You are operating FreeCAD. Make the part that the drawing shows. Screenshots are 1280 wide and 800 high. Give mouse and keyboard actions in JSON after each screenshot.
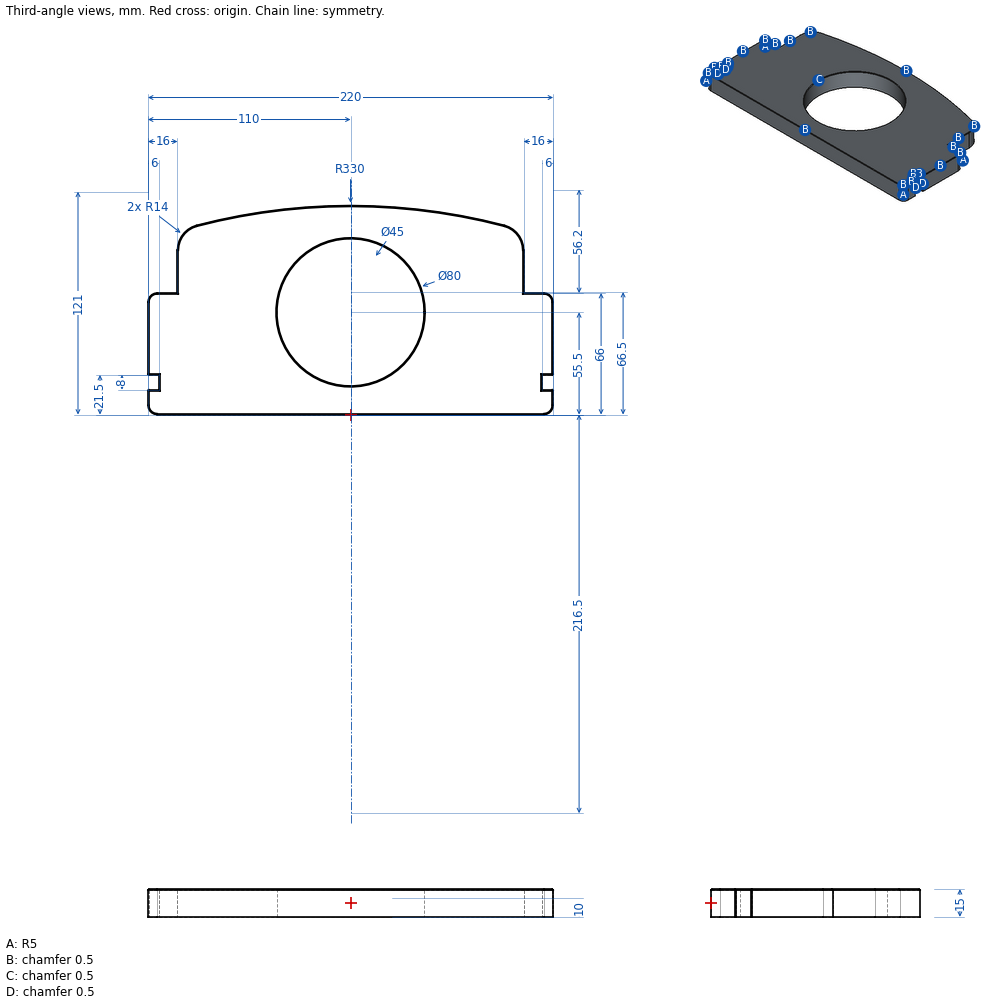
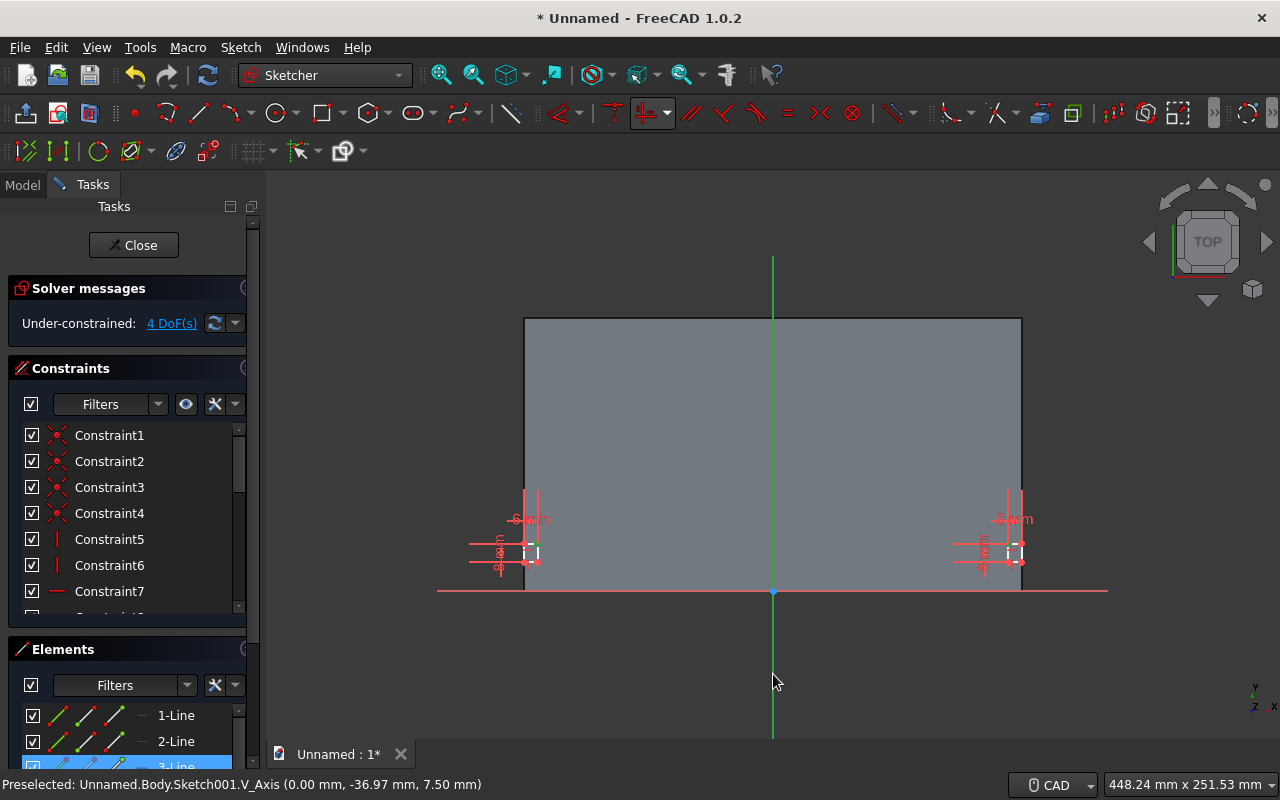
{"action": "left_click", "coordinate": [820, 114]}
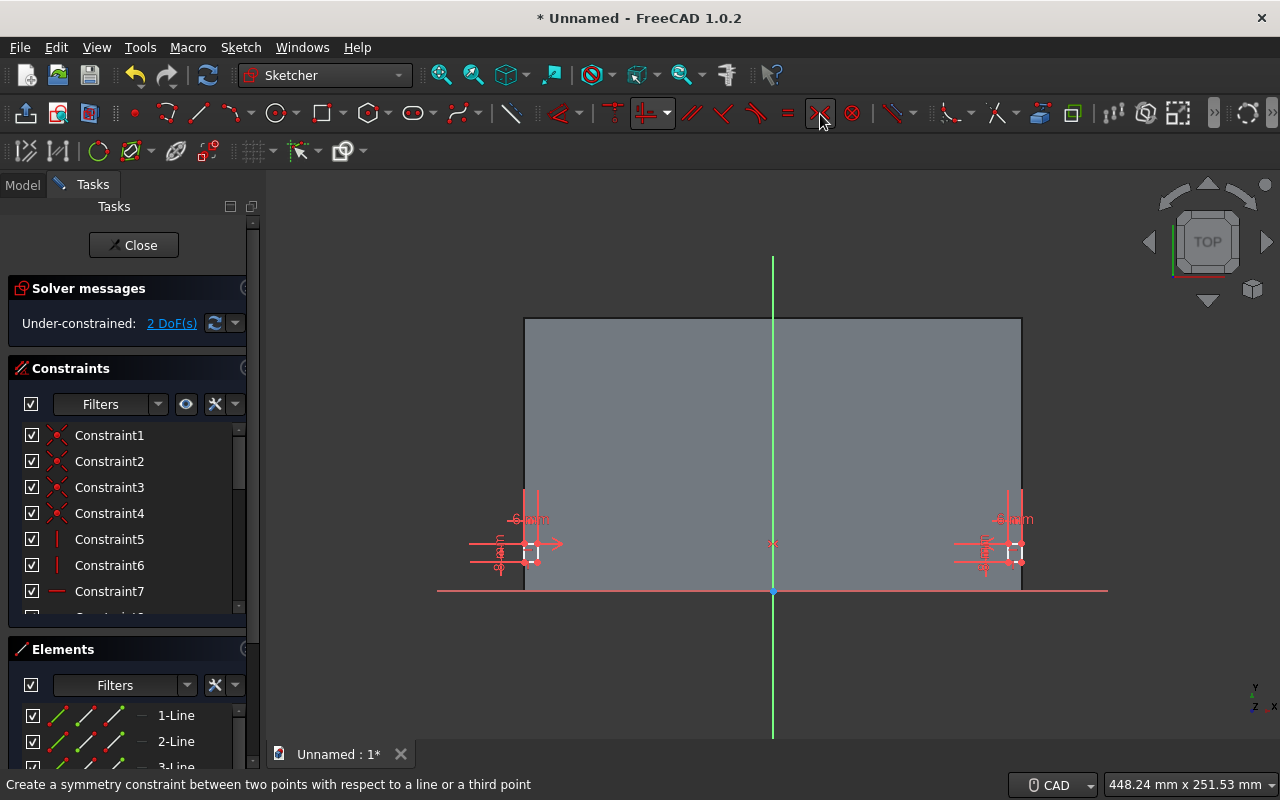
{"action": "left_click", "coordinate": [558, 114]}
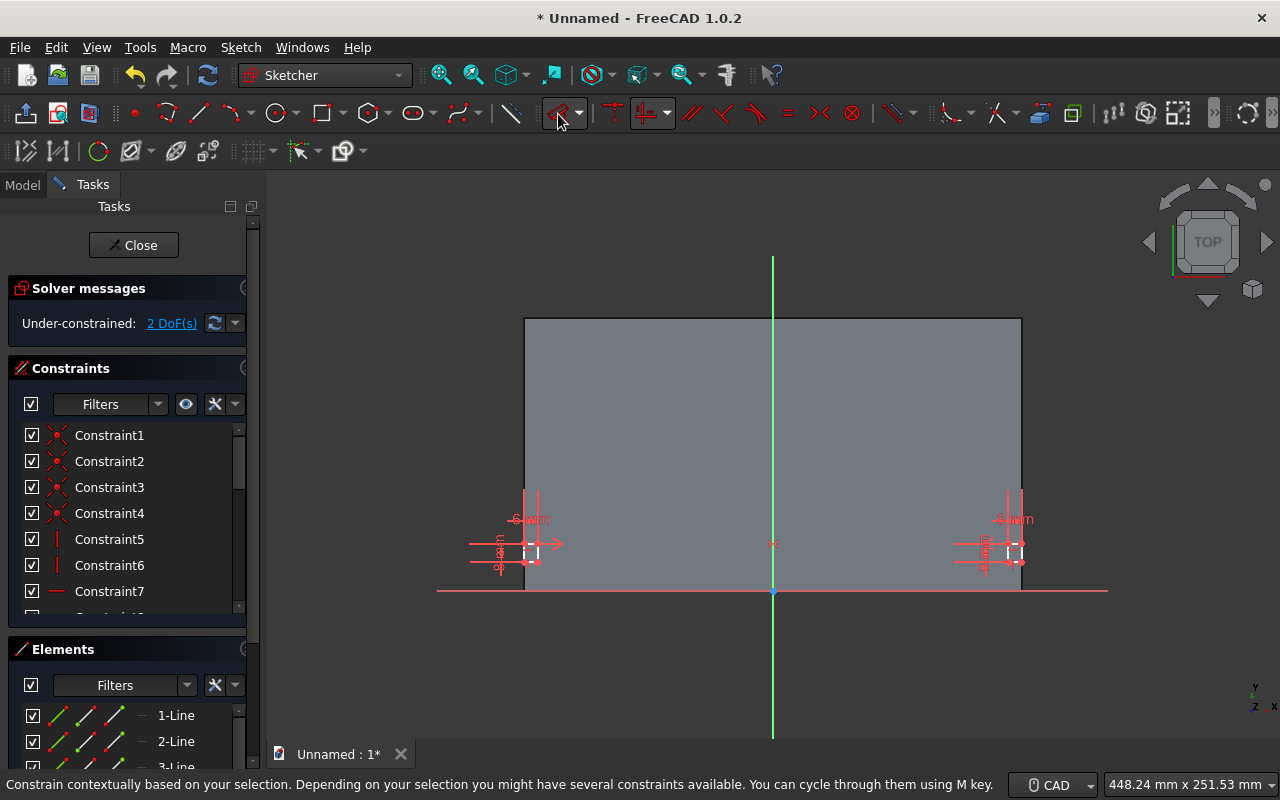
{"action": "left_click", "coordinate": [524, 544]}
{"action": "left_click", "coordinate": [649, 625]}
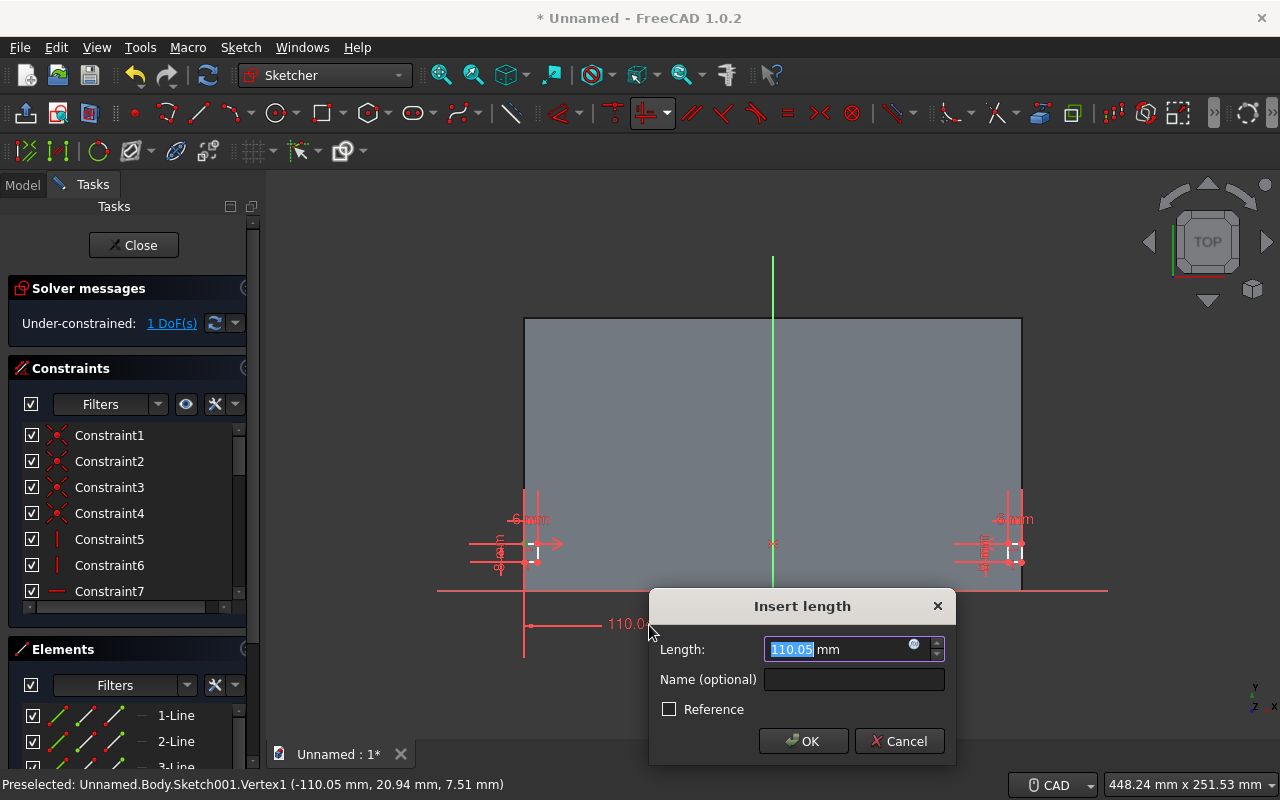
{"action": "type", "text": "110"}
{"action": "key", "text": "Return"}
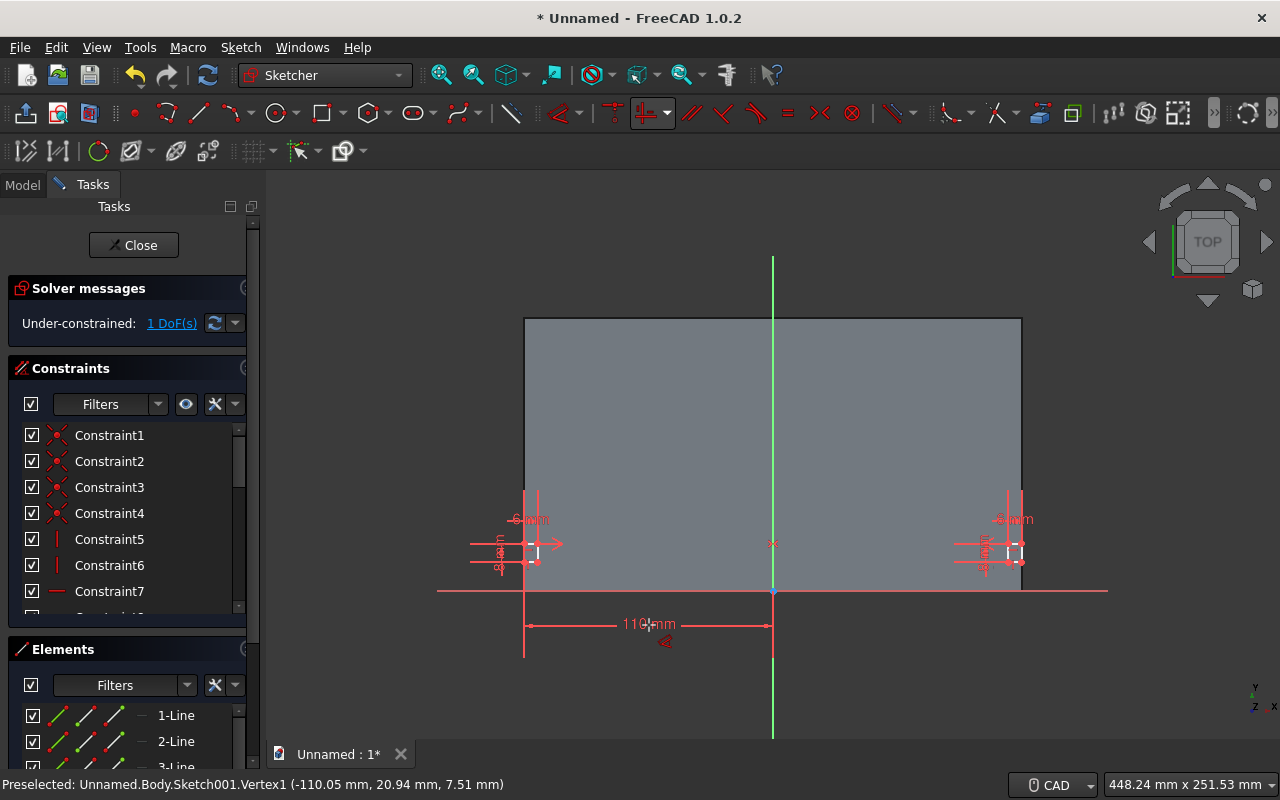
{"action": "left_click", "coordinate": [524, 544]}
{"action": "left_click", "coordinate": [490, 568]}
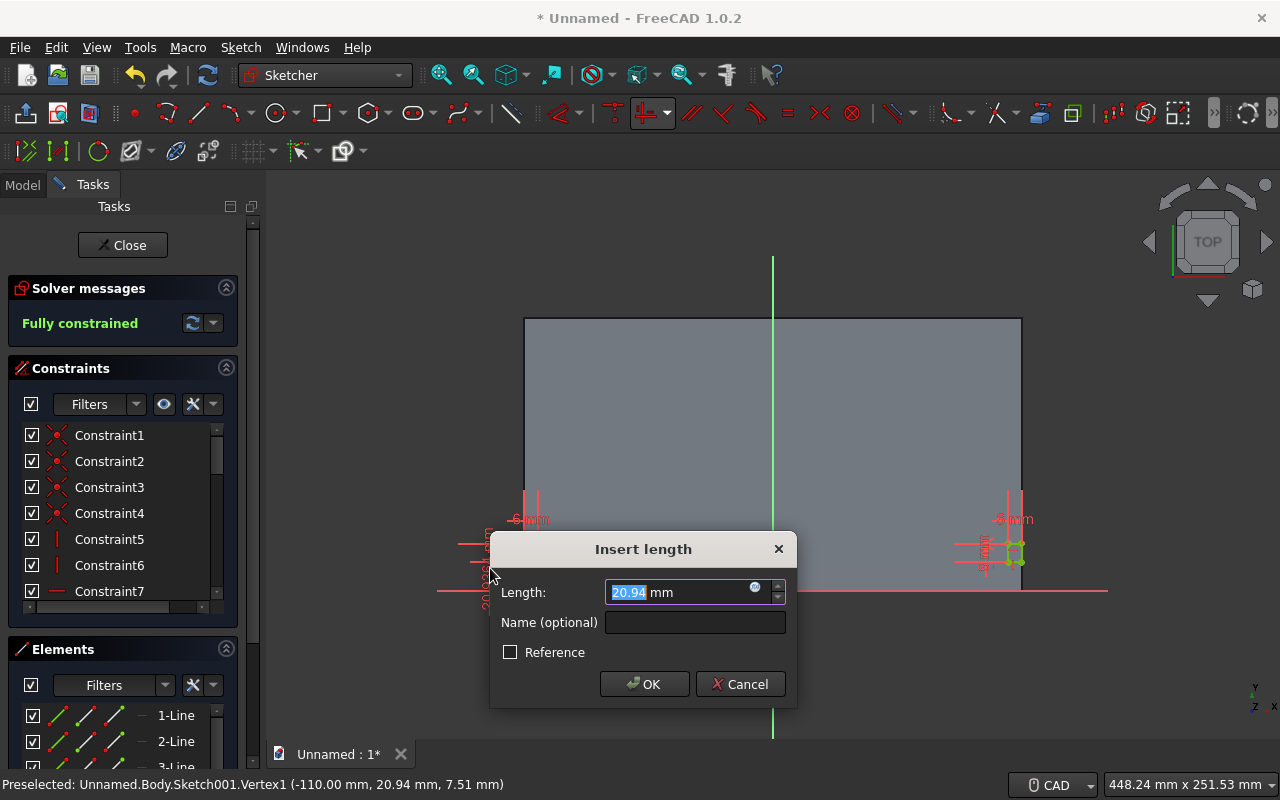
{"action": "type", "text": "21.5"}
{"action": "key", "text": "Return"}
{"action": "key", "text": "Escape"}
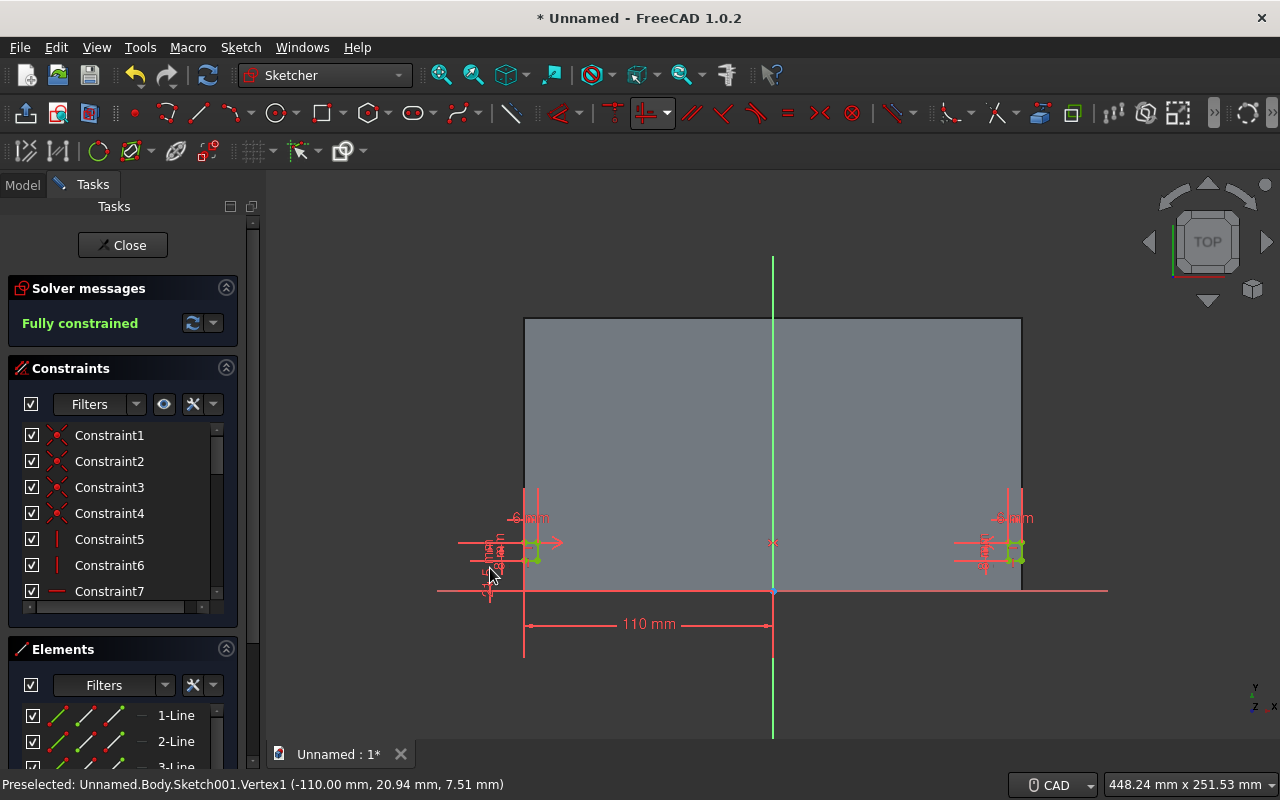
{"action": "left_click", "coordinate": [123, 245]}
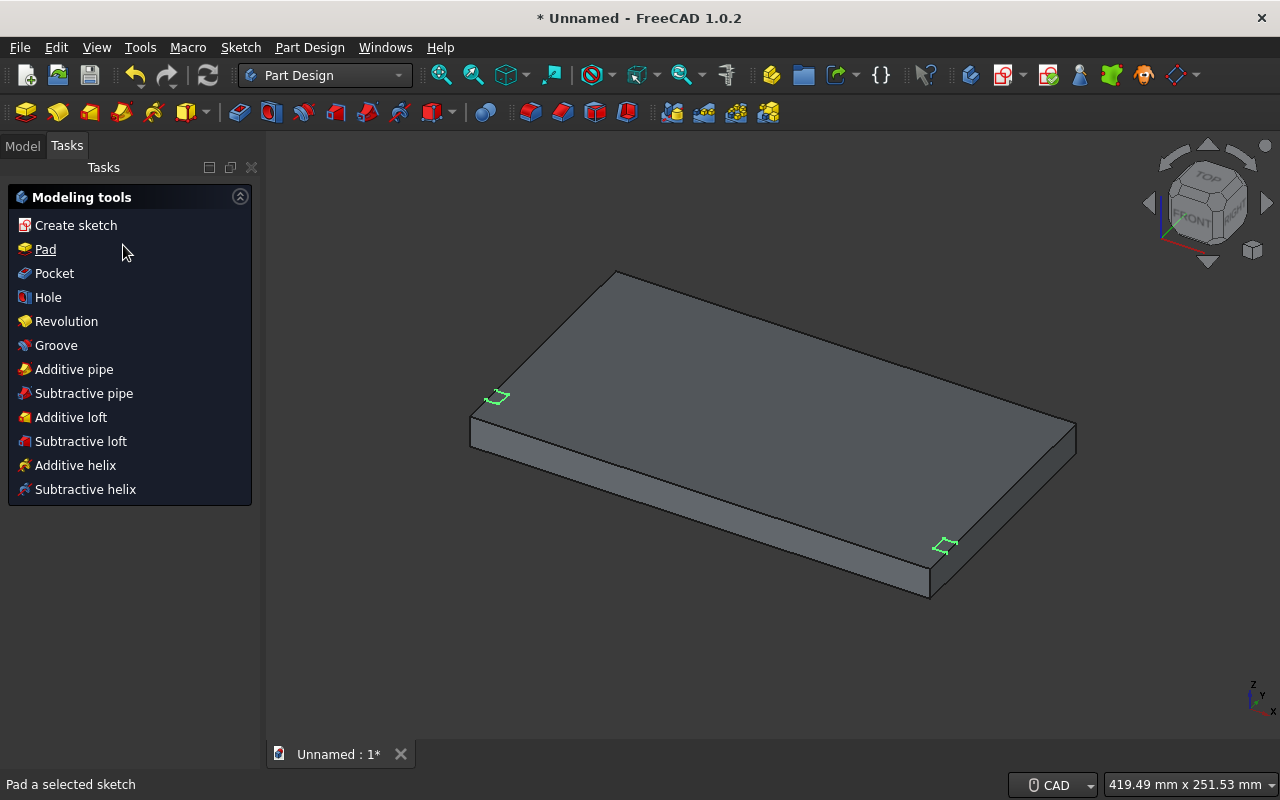
{"action": "left_click", "coordinate": [240, 112]}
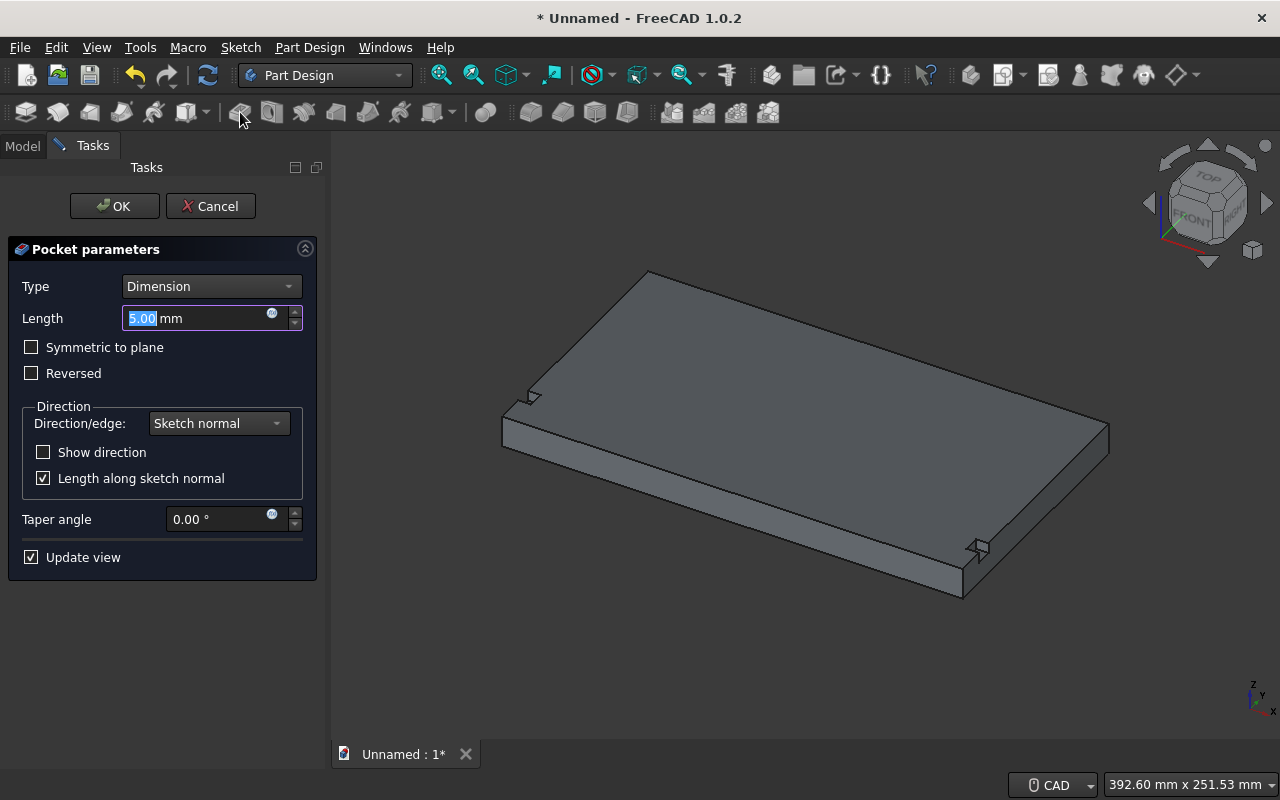
{"action": "left_click", "coordinate": [212, 286]}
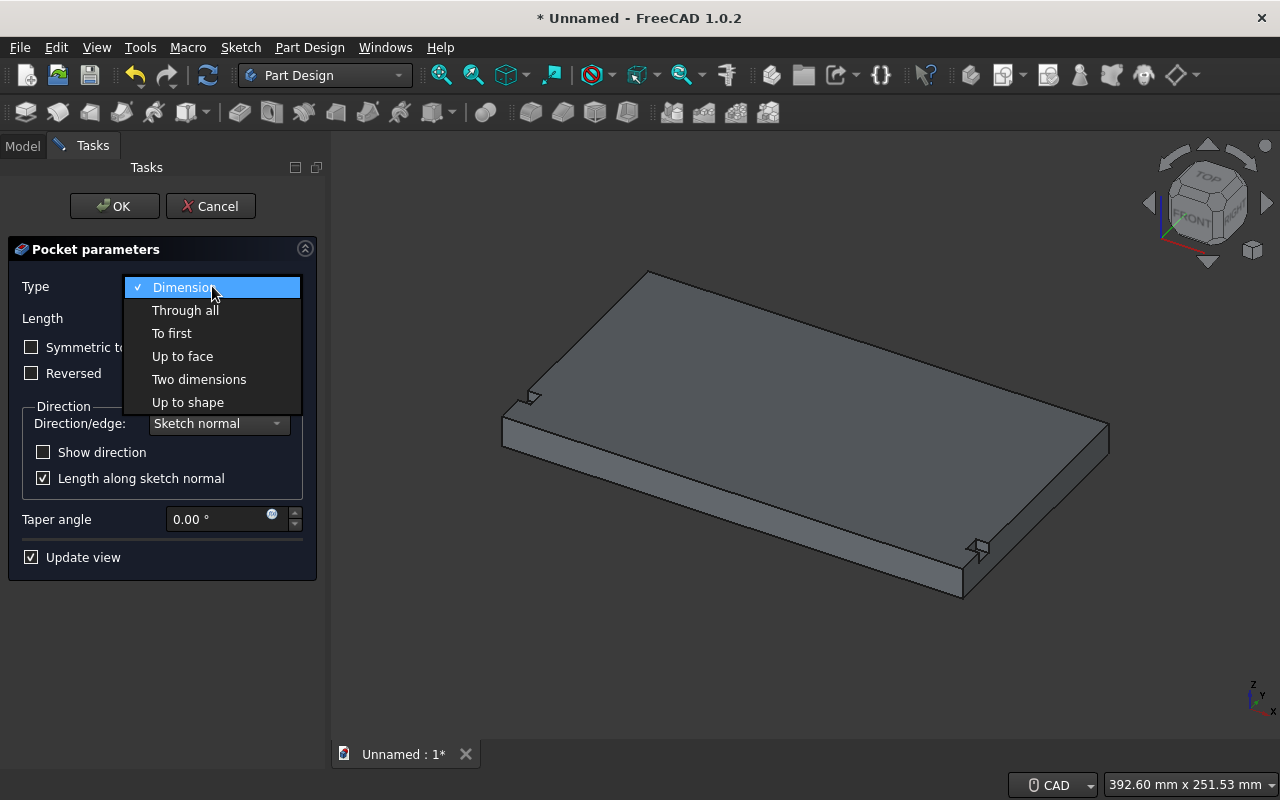
{"action": "left_click", "coordinate": [212, 310]}